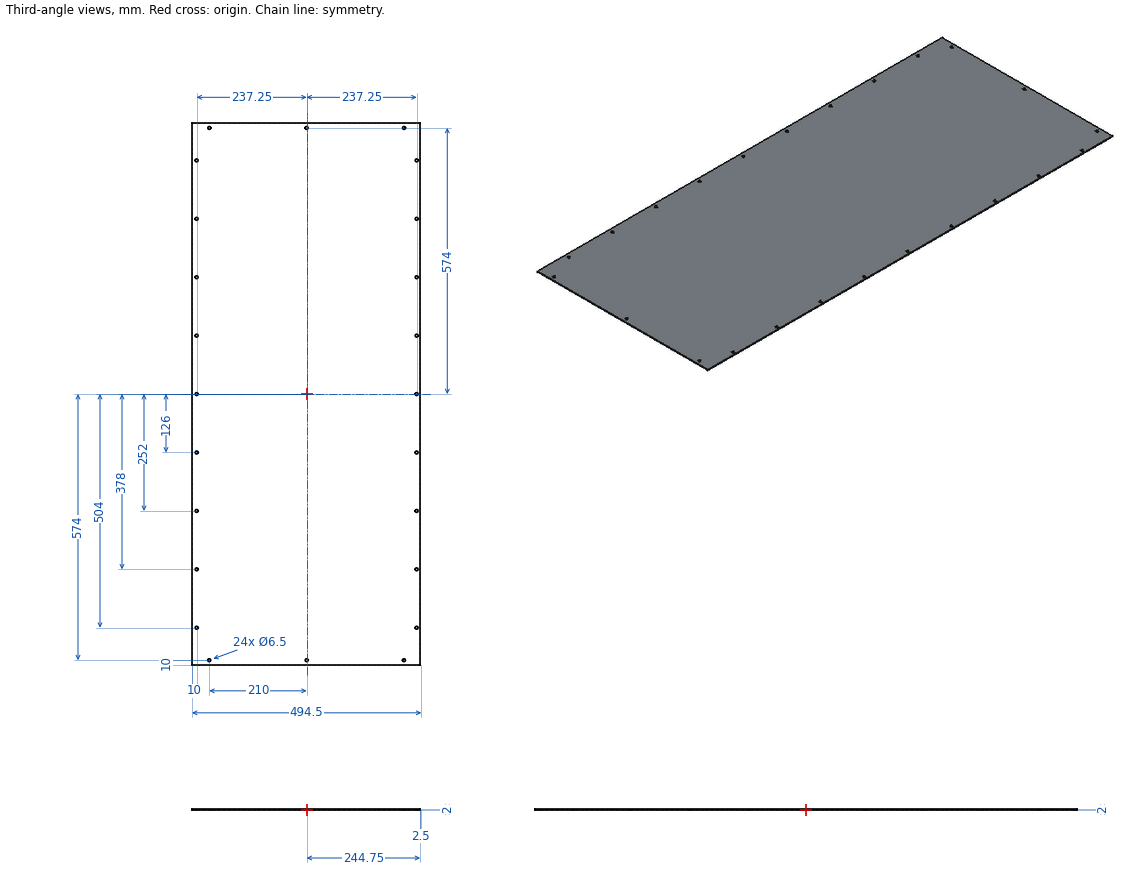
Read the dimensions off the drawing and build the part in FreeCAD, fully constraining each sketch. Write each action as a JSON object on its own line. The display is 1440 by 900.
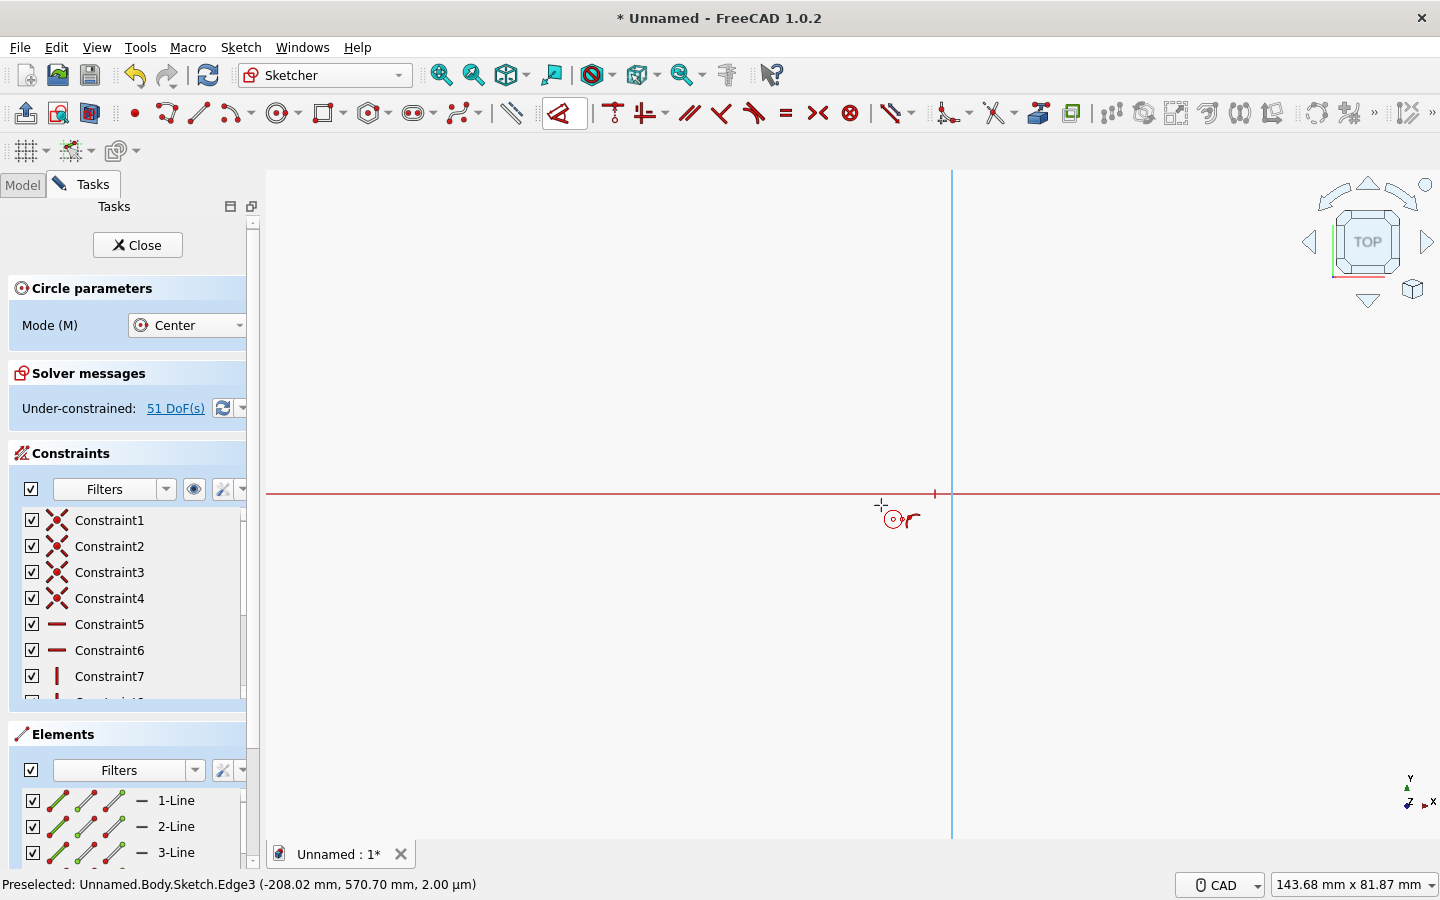
{"action": "scroll", "coordinate": [881, 505], "scroll_direction": "down", "scroll_amount": 15}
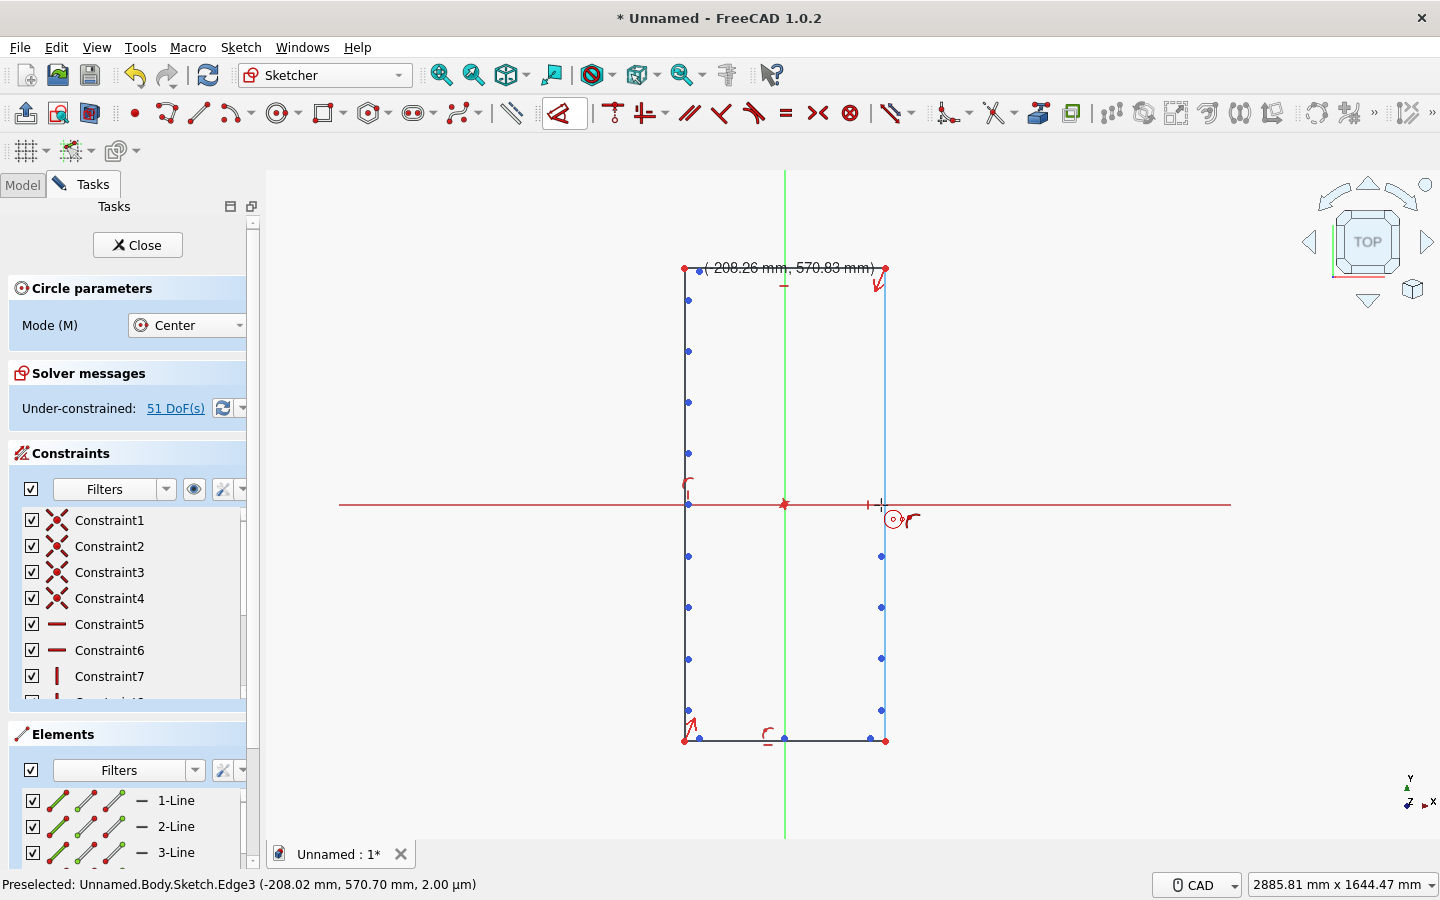
{"action": "scroll", "coordinate": [881, 505], "scroll_direction": "up", "scroll_amount": 7}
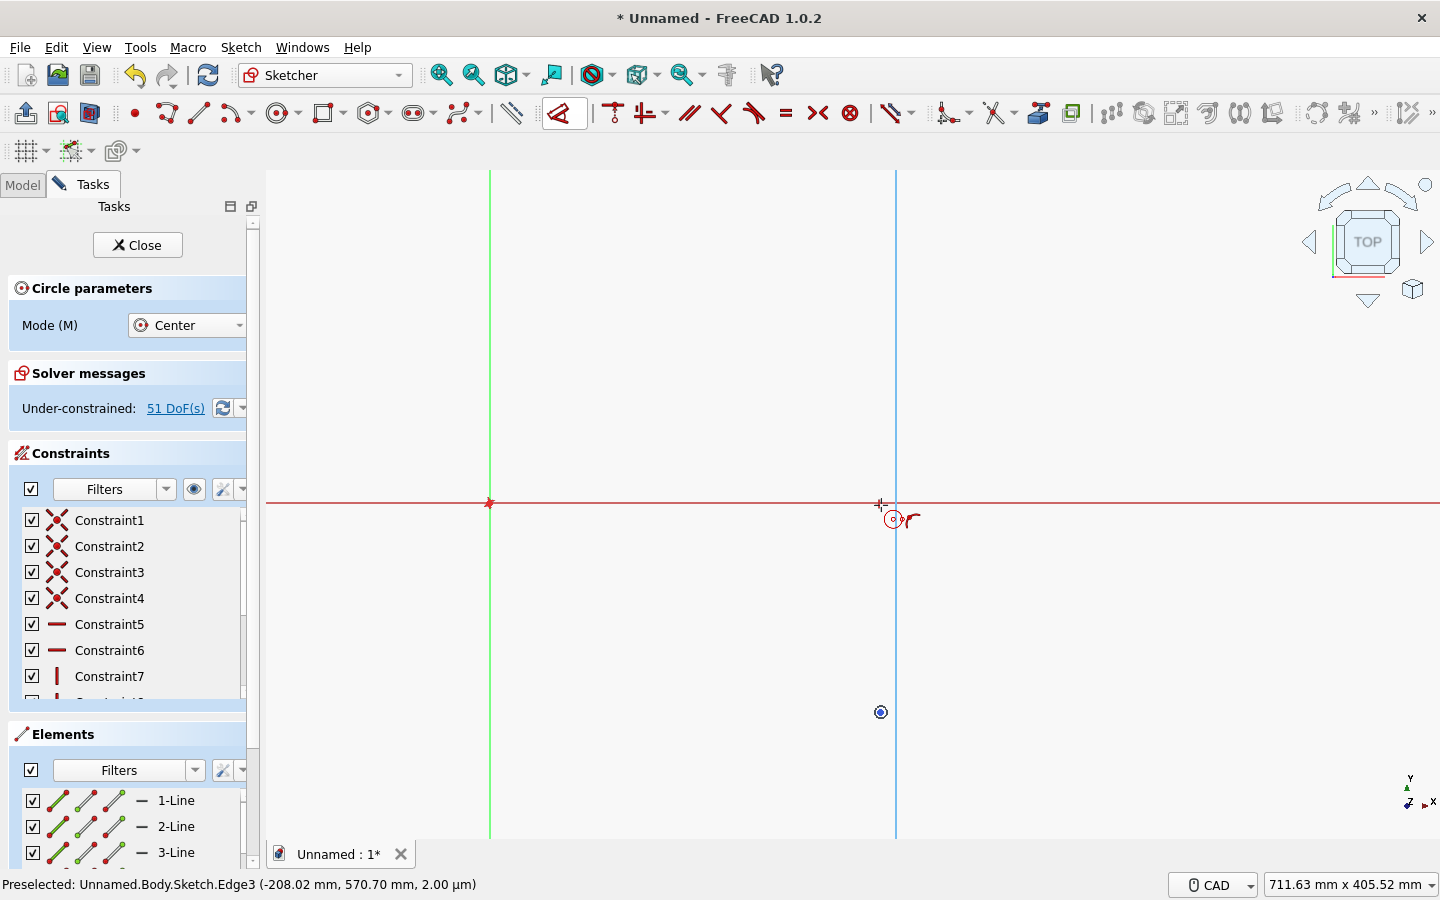
{"action": "left_click", "coordinate": [881, 503]}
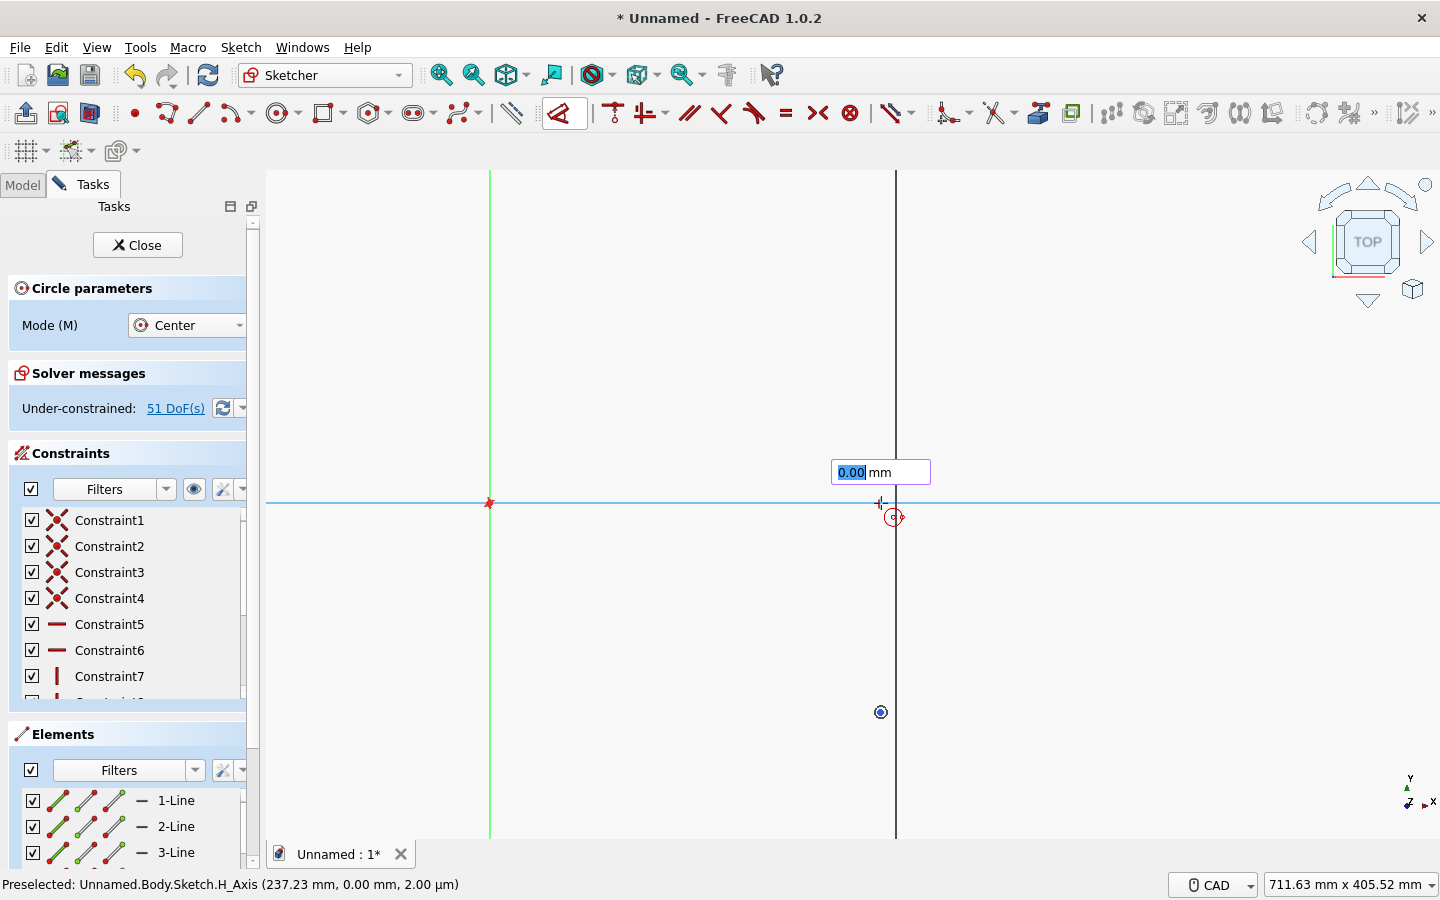
{"action": "scroll", "coordinate": [879, 508], "scroll_direction": "up", "scroll_amount": 6}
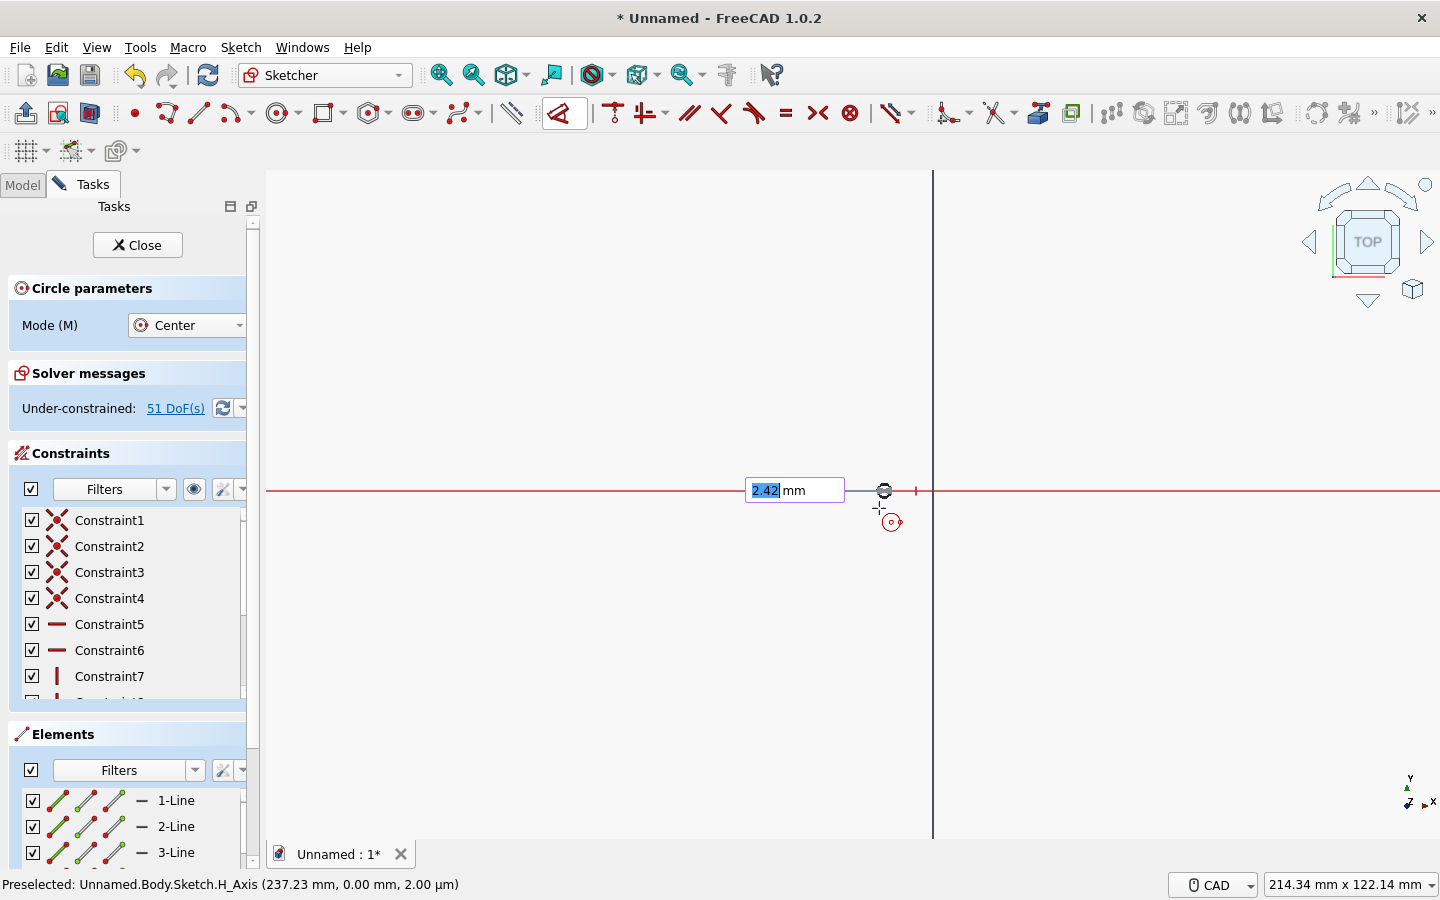
{"action": "left_click", "coordinate": [878, 507]}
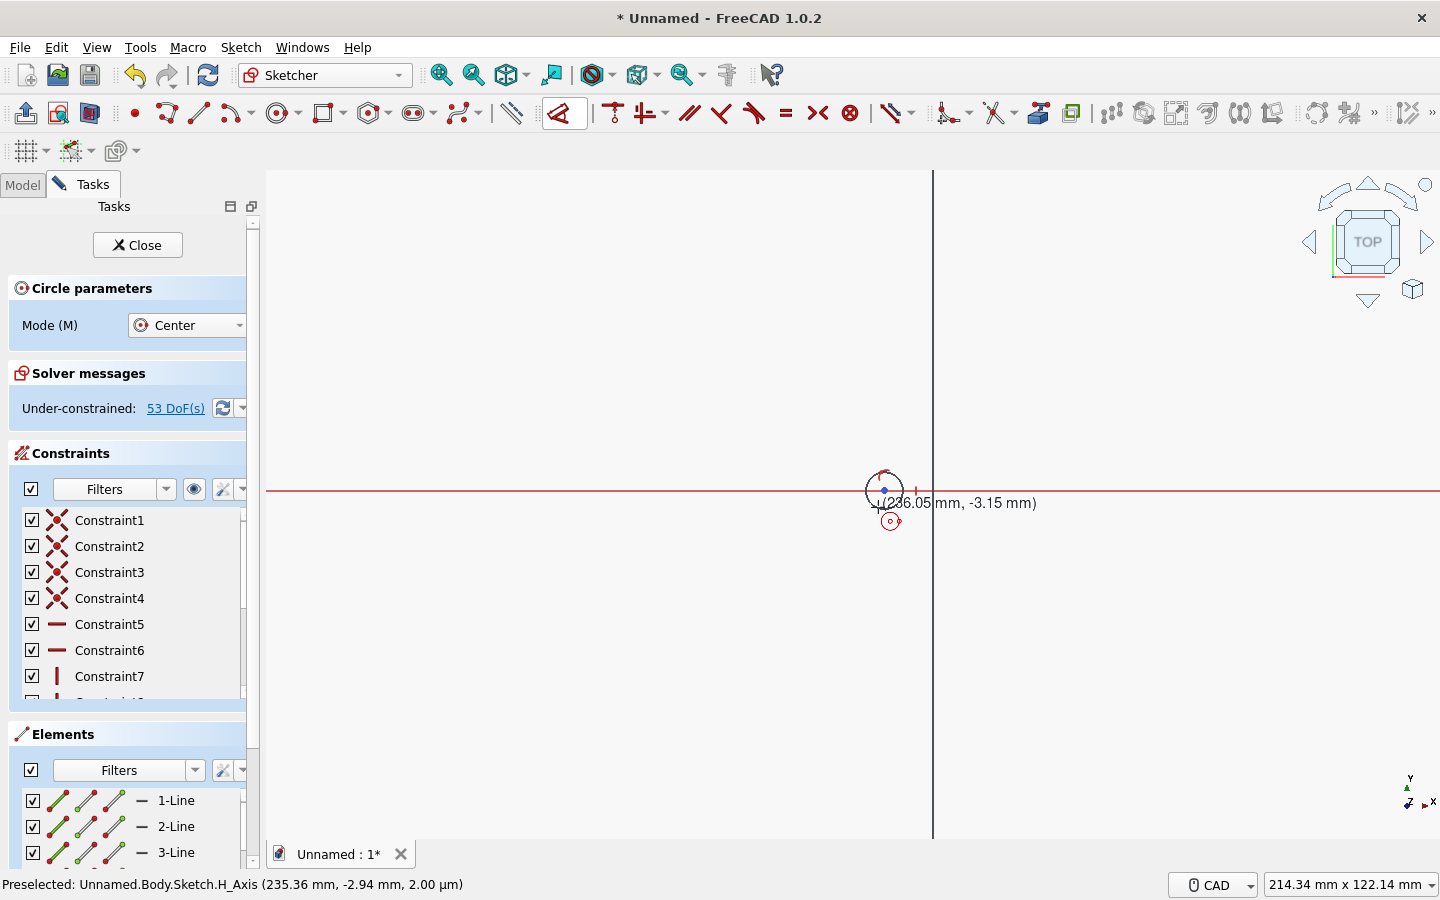
{"action": "scroll", "coordinate": [881, 506], "scroll_direction": "down", "scroll_amount": 13}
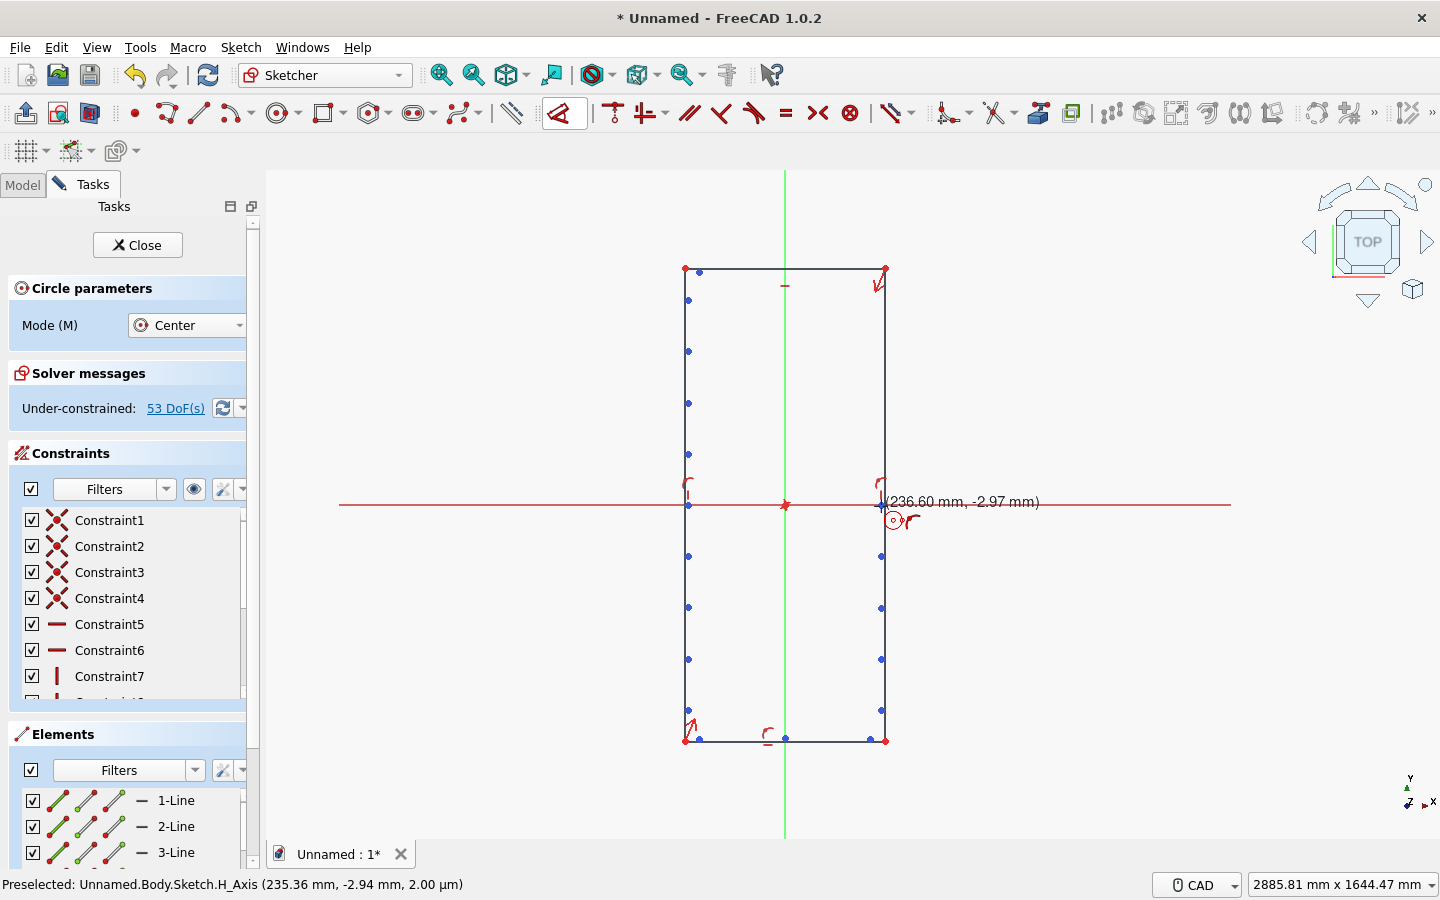
{"action": "scroll", "coordinate": [882, 454], "scroll_direction": "up", "scroll_amount": 15}